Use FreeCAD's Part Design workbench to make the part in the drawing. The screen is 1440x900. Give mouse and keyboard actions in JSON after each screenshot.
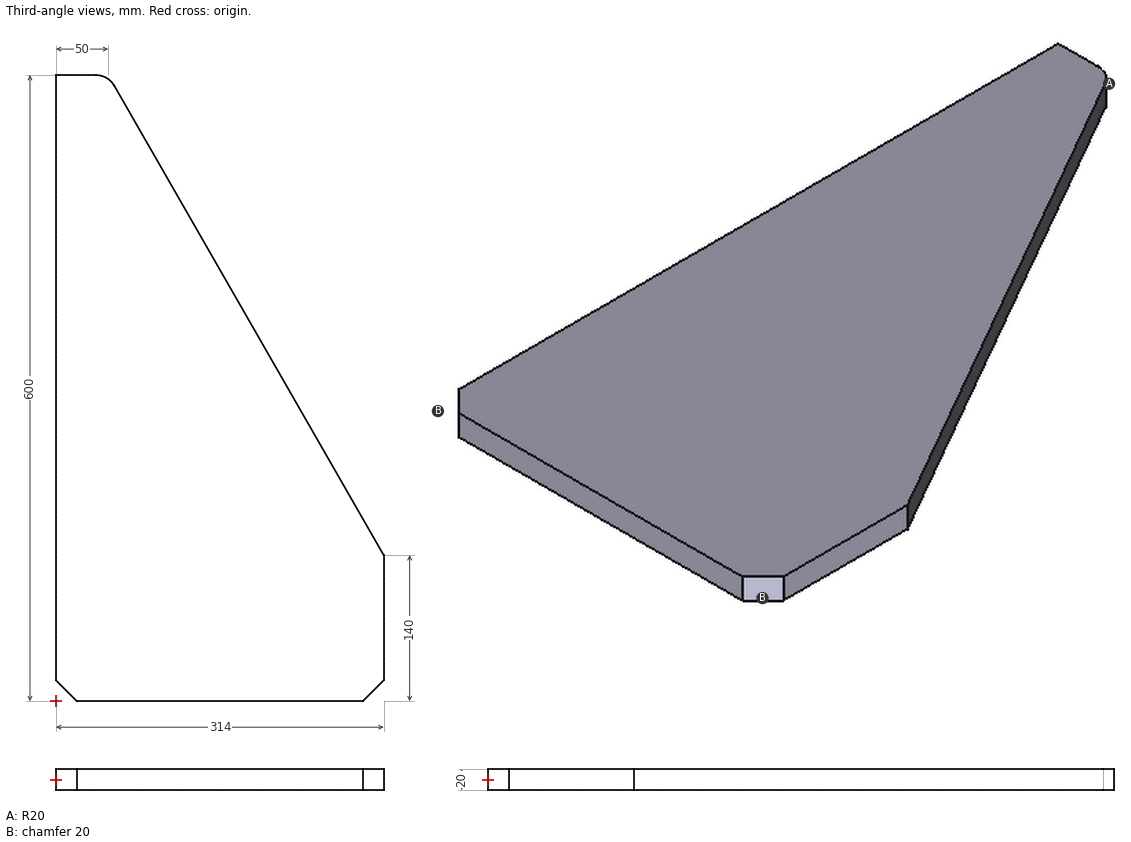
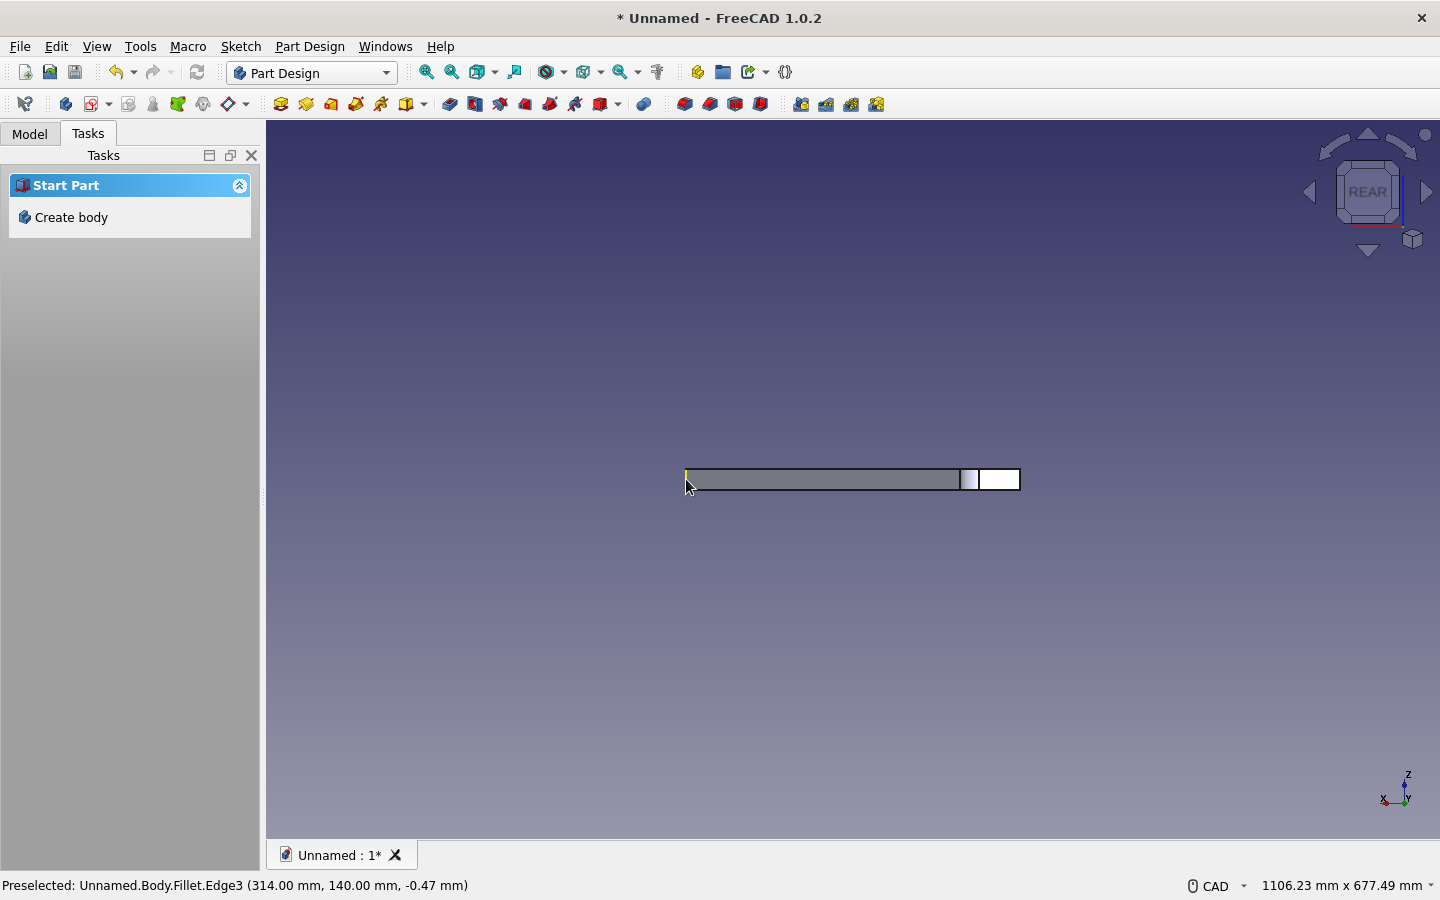
{"action": "key", "text": "0"}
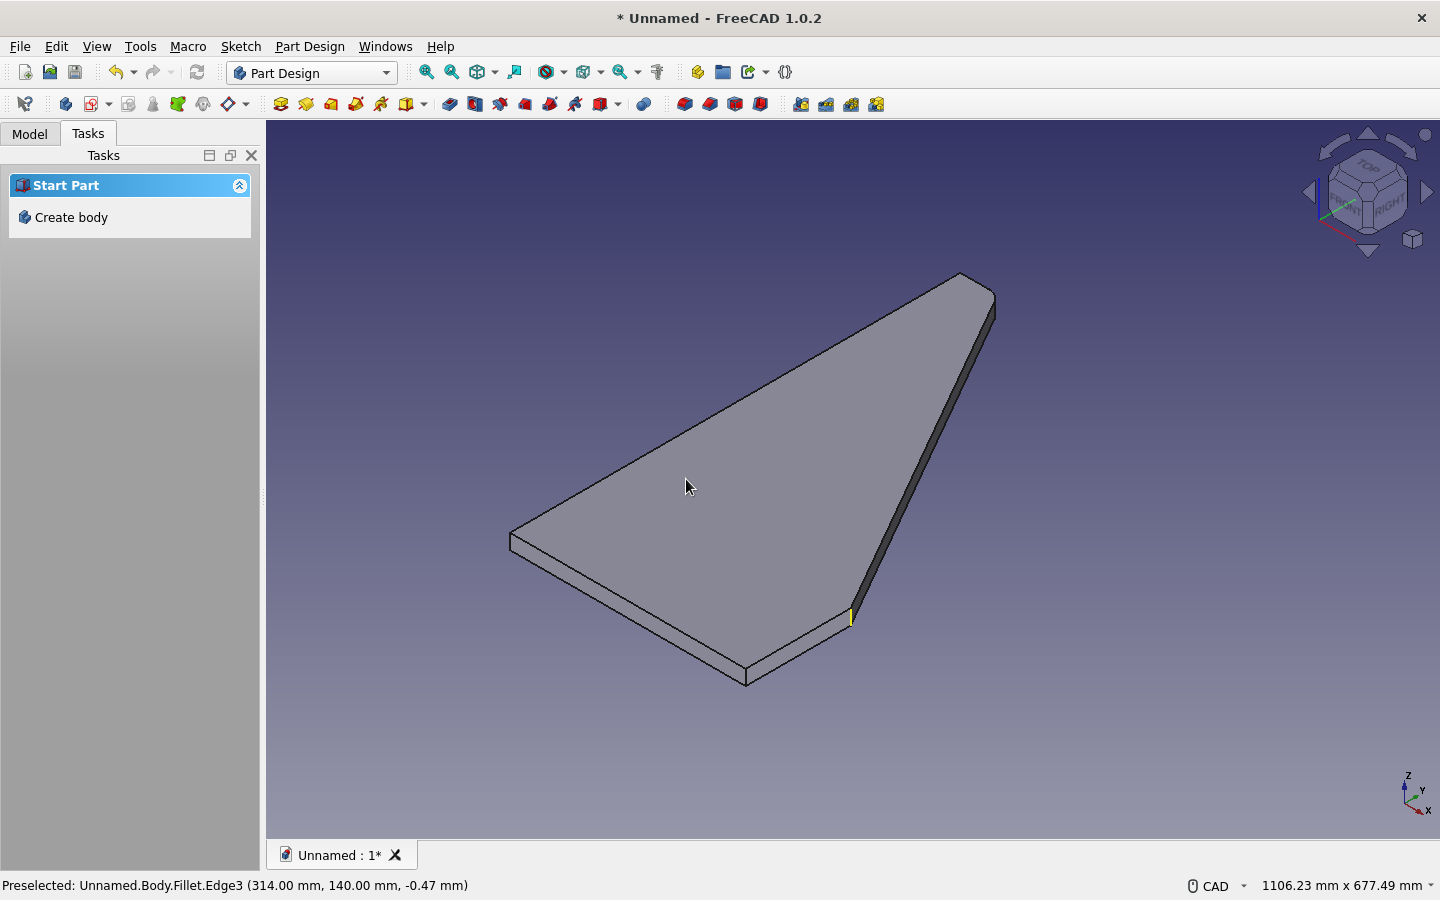
{"action": "left_click", "coordinate": [746, 676]}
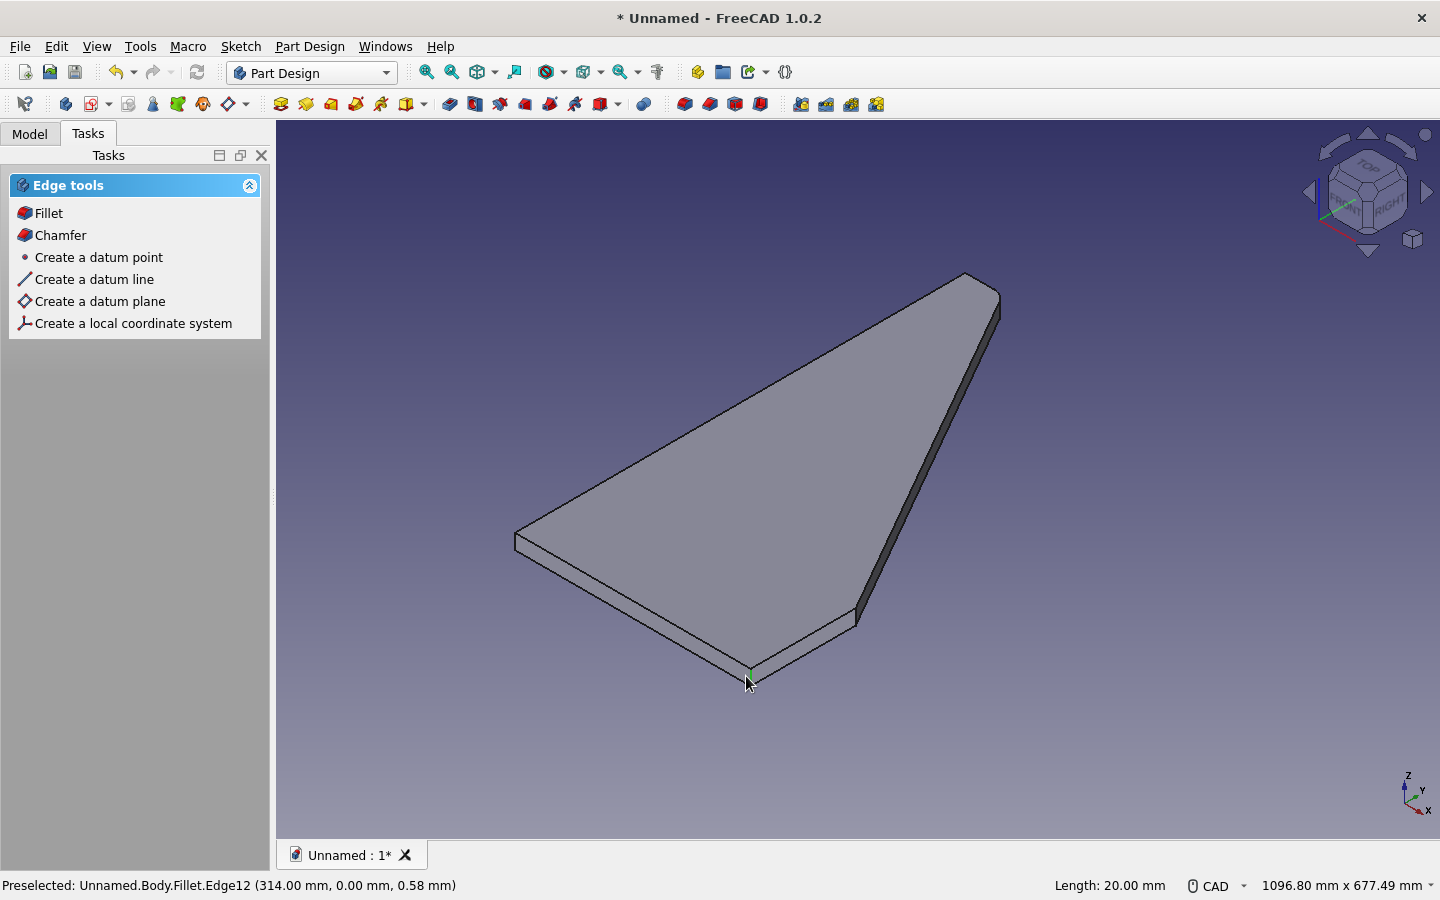
{"action": "scroll", "coordinate": [515, 540], "scroll_direction": "up", "scroll_amount": 4}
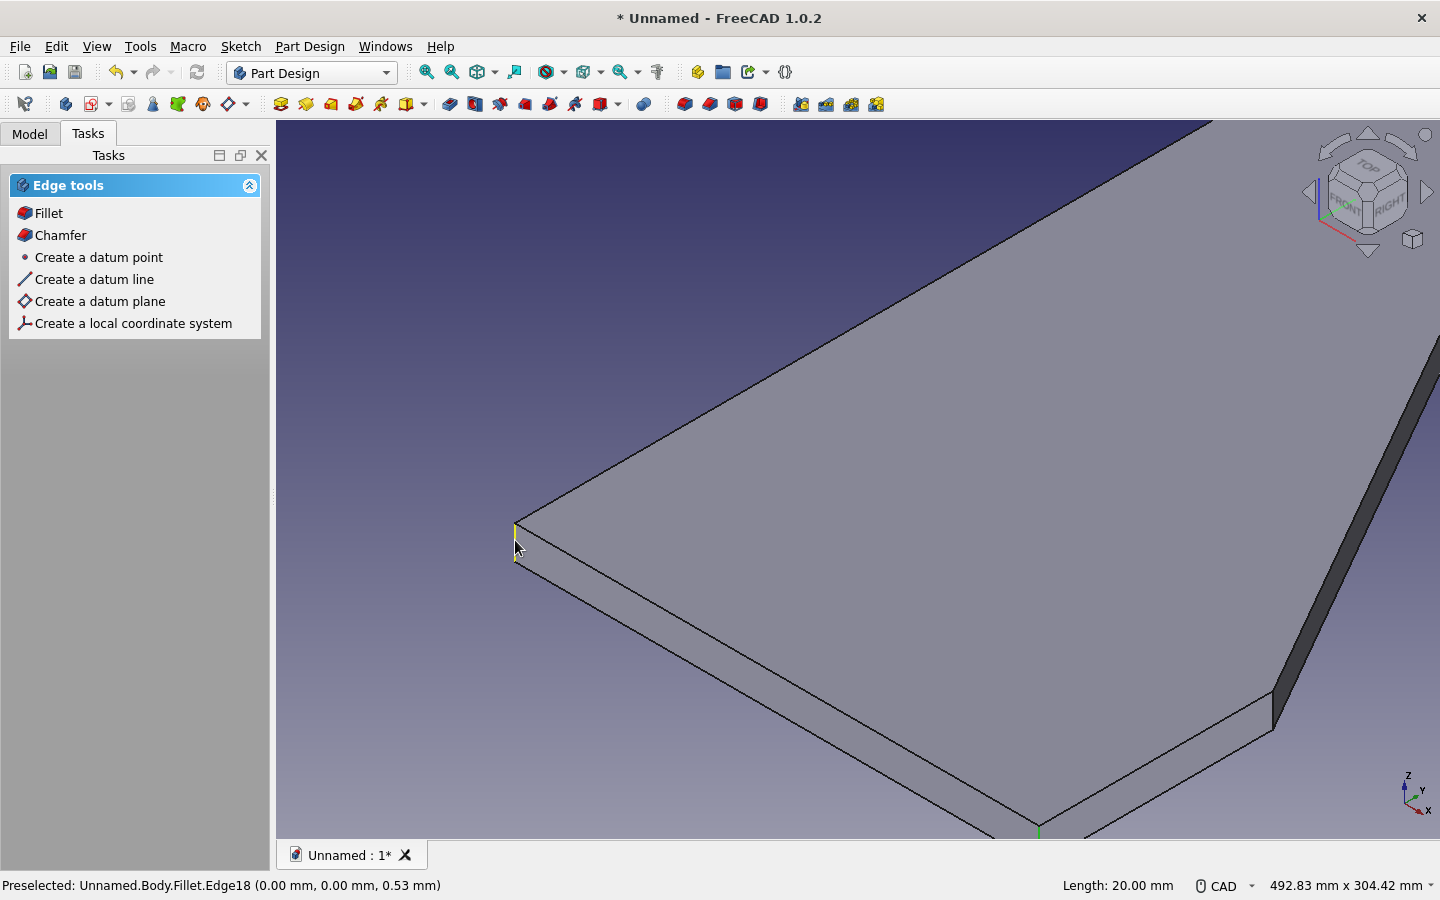
{"action": "left_click", "coordinate": [427, 72]}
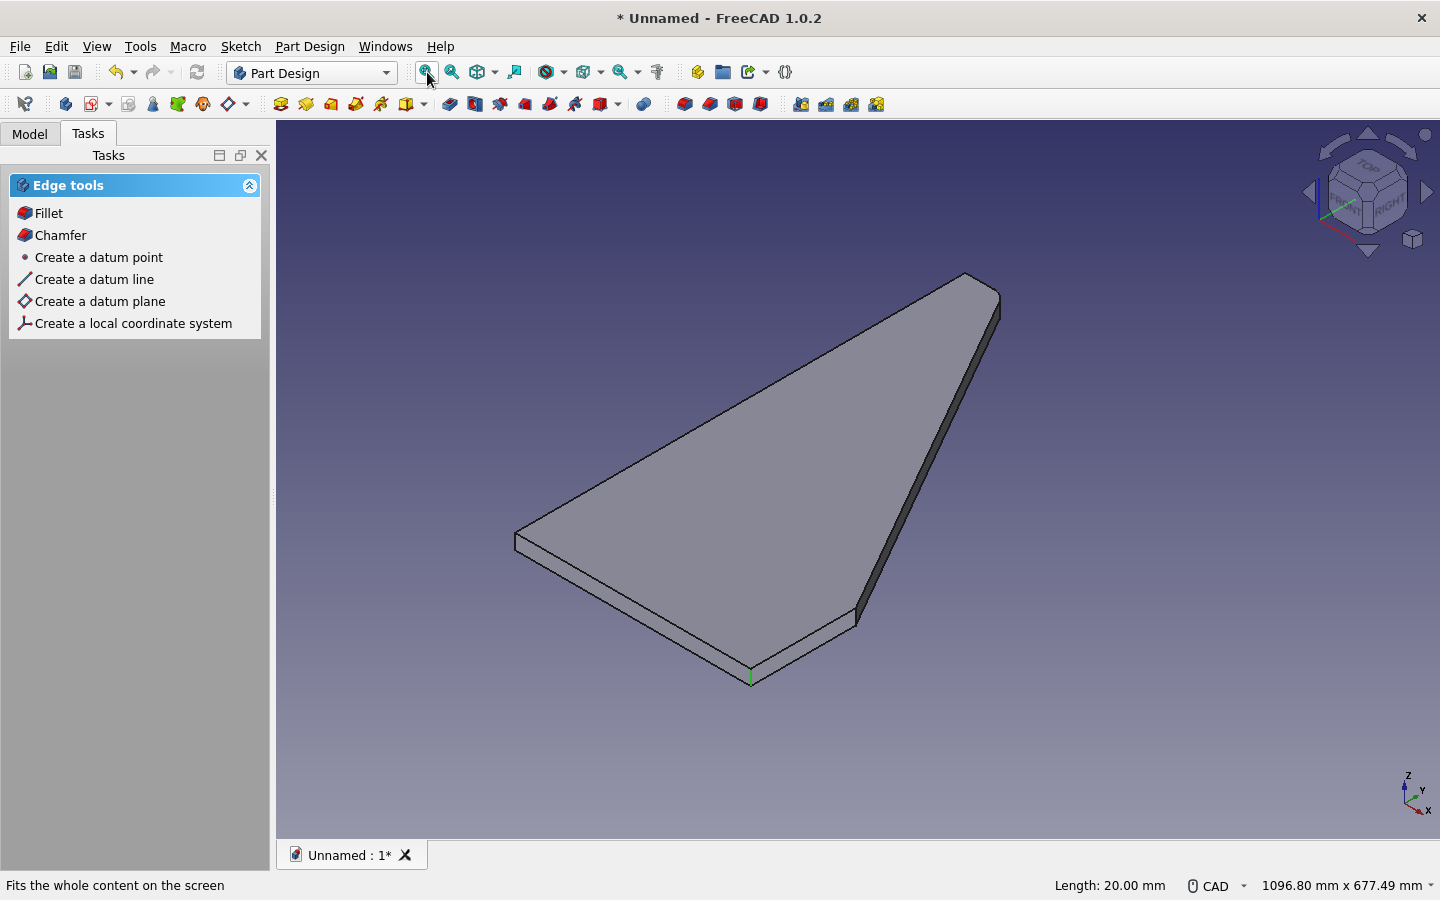
{"action": "key", "text": "2"}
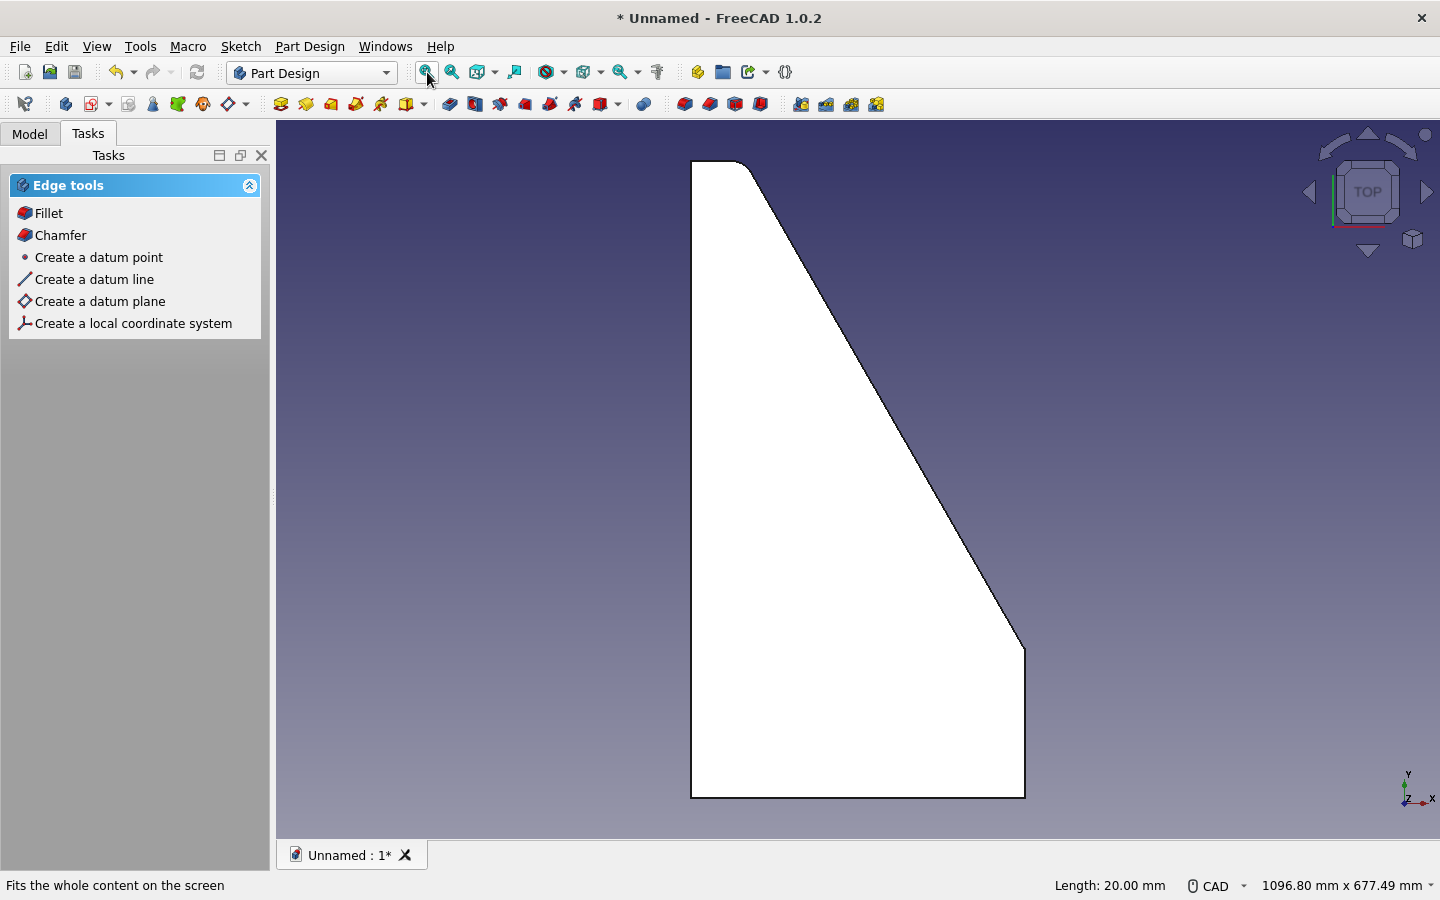
{"action": "scroll", "coordinate": [691, 797], "scroll_direction": "up", "scroll_amount": 4}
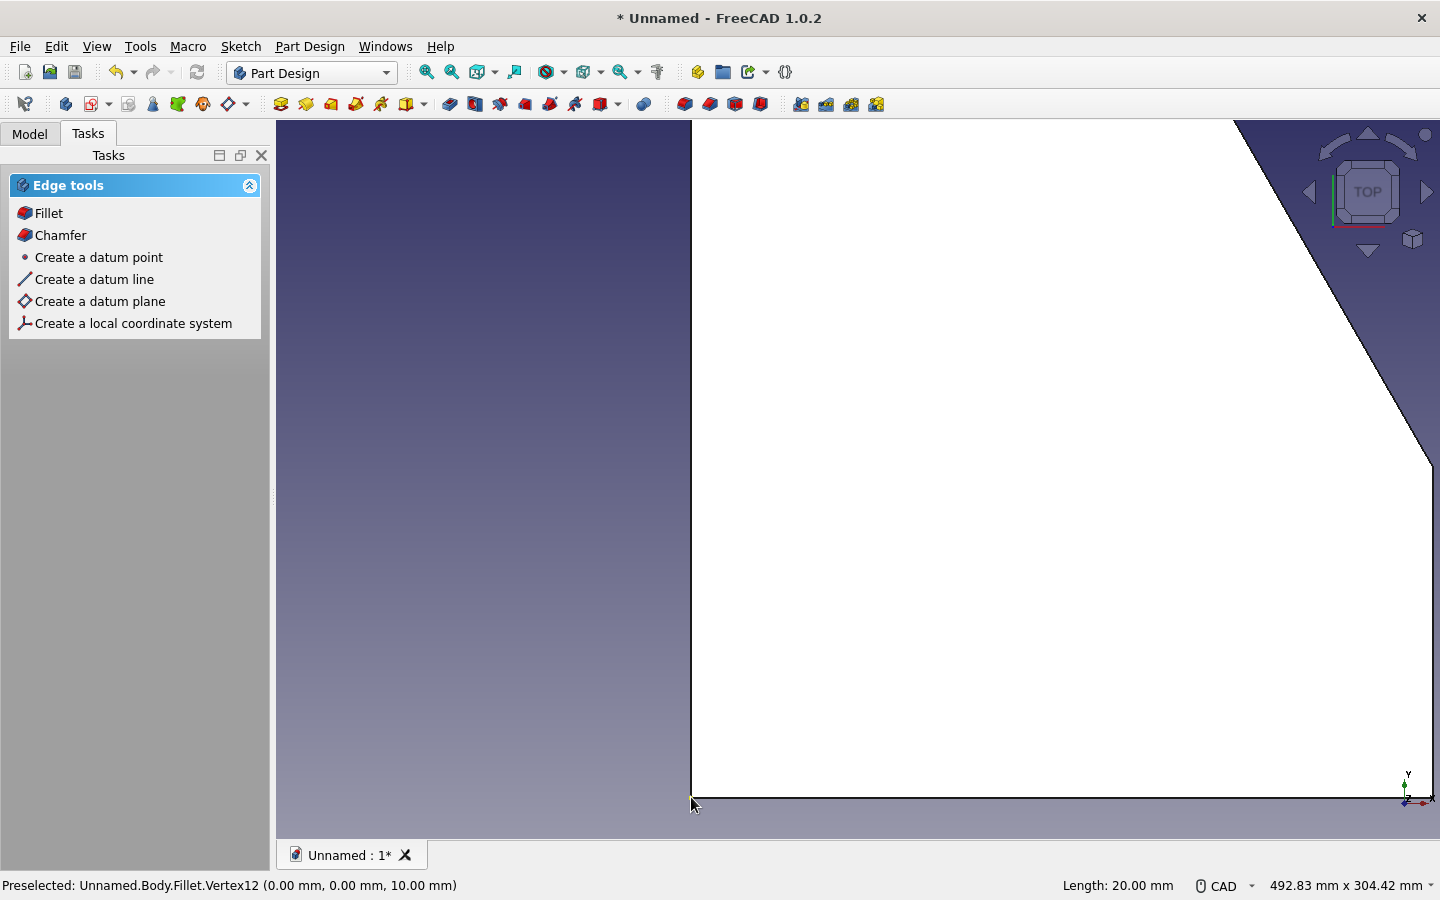
{"action": "left_click", "coordinate": [427, 72]}